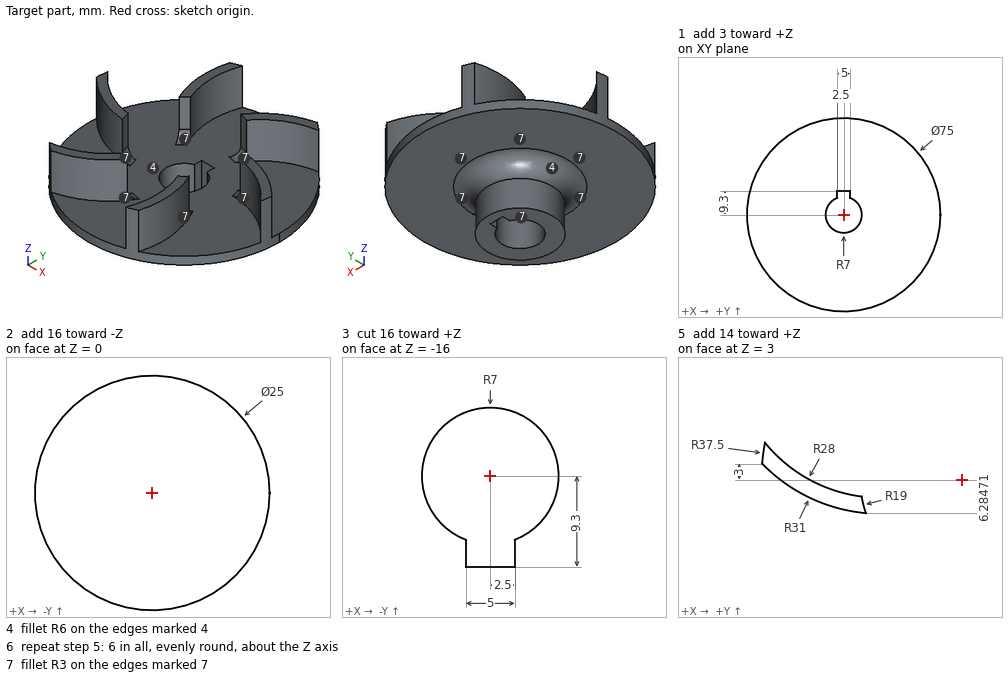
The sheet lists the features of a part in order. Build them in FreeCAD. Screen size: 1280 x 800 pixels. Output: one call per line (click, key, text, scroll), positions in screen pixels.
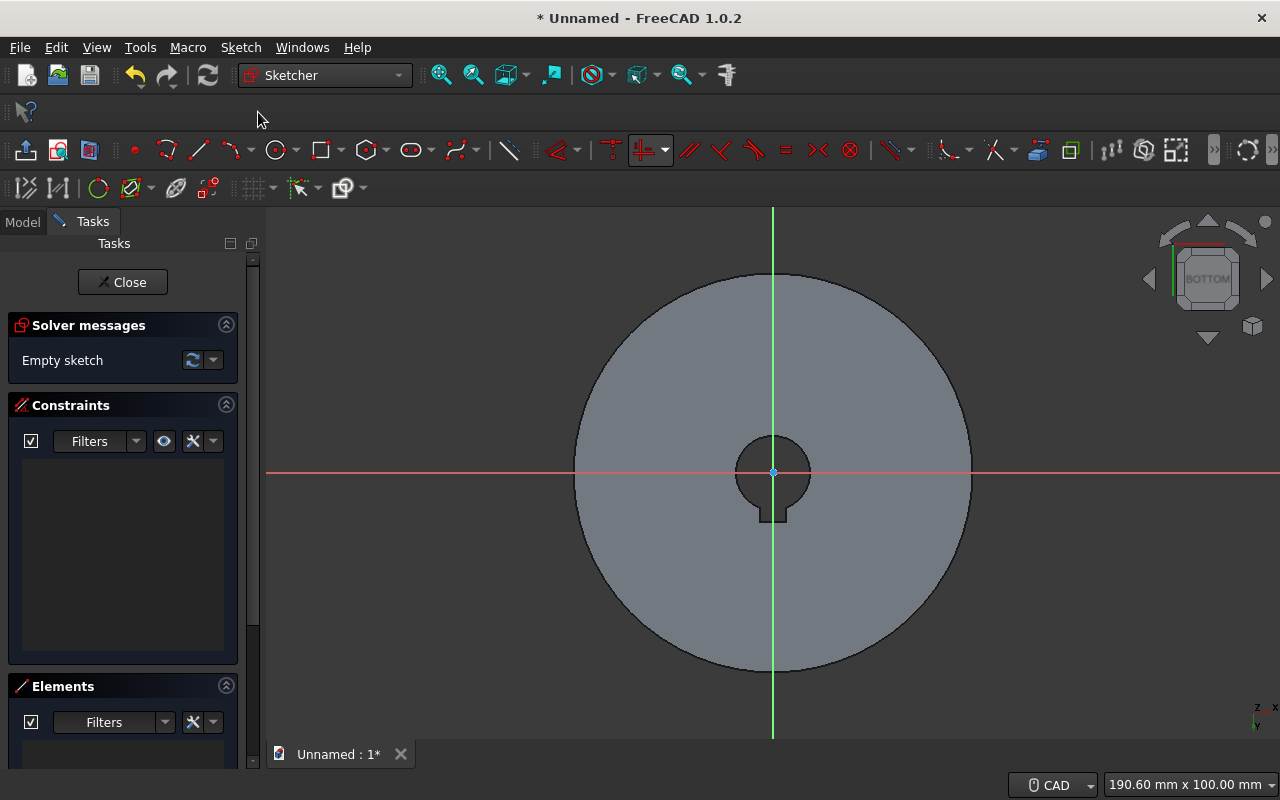
scroll(813, 473, up, 5)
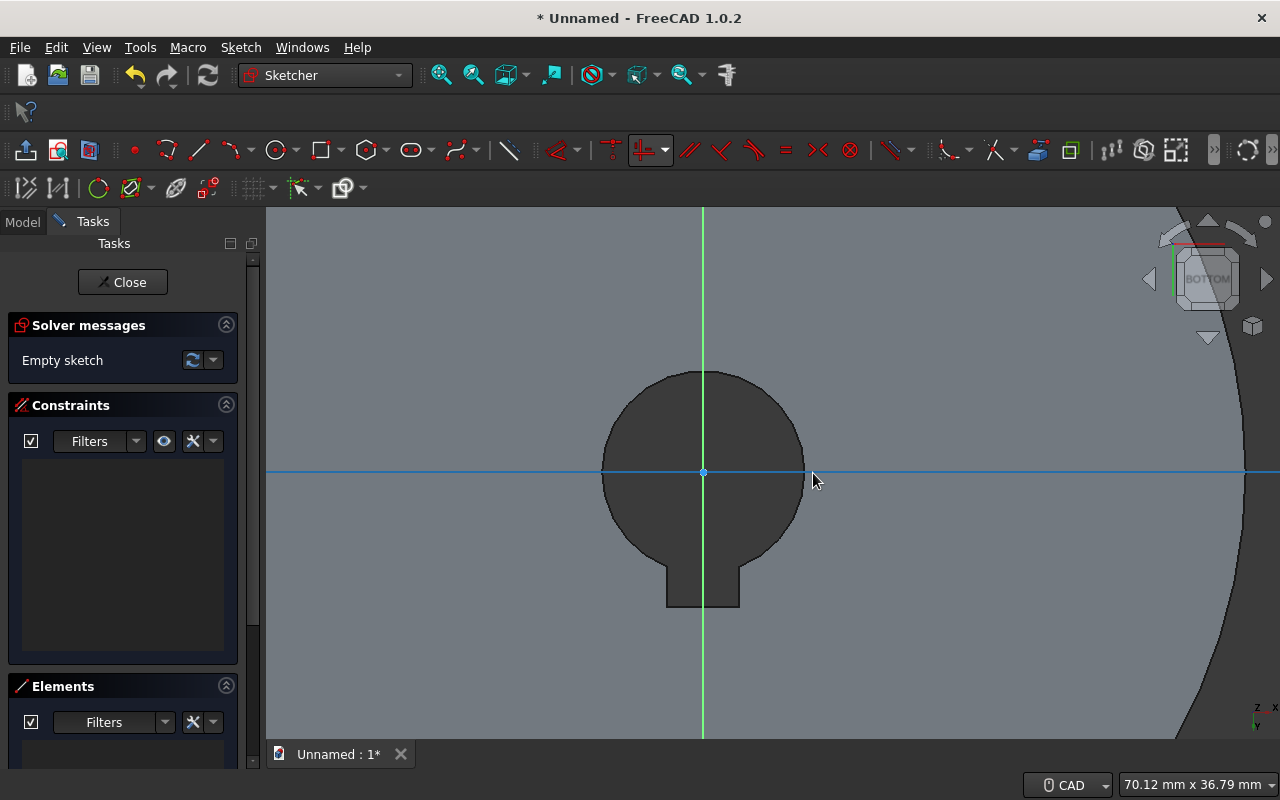
click(276, 150)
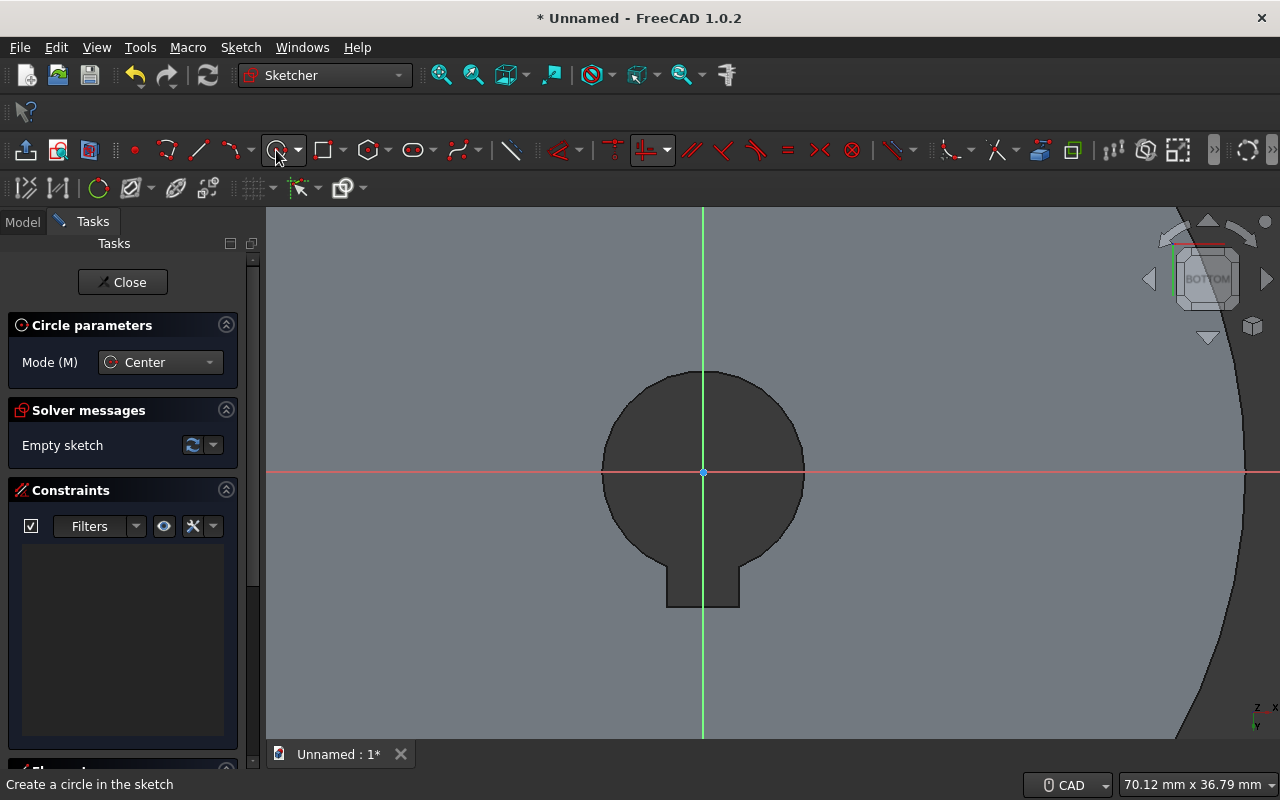
click(703, 472)
click(831, 344)
key(Escape)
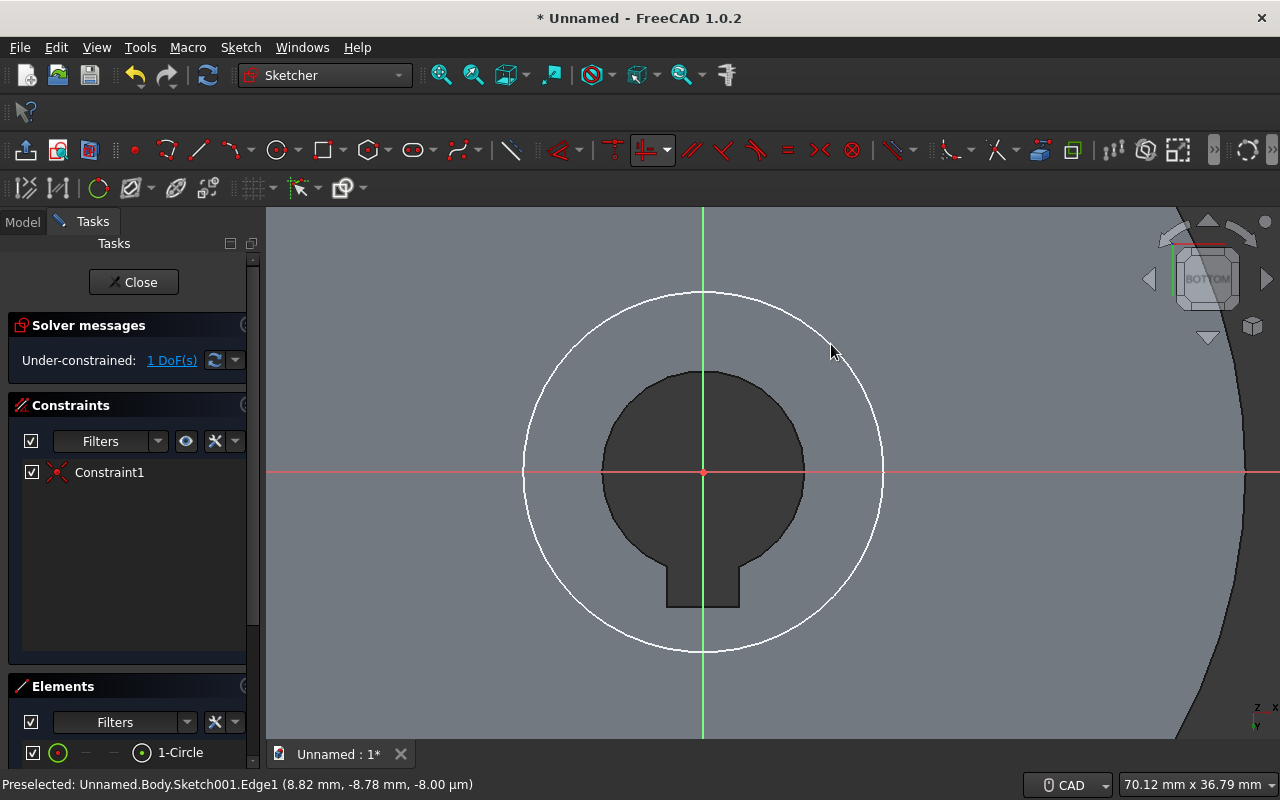
click(830, 344)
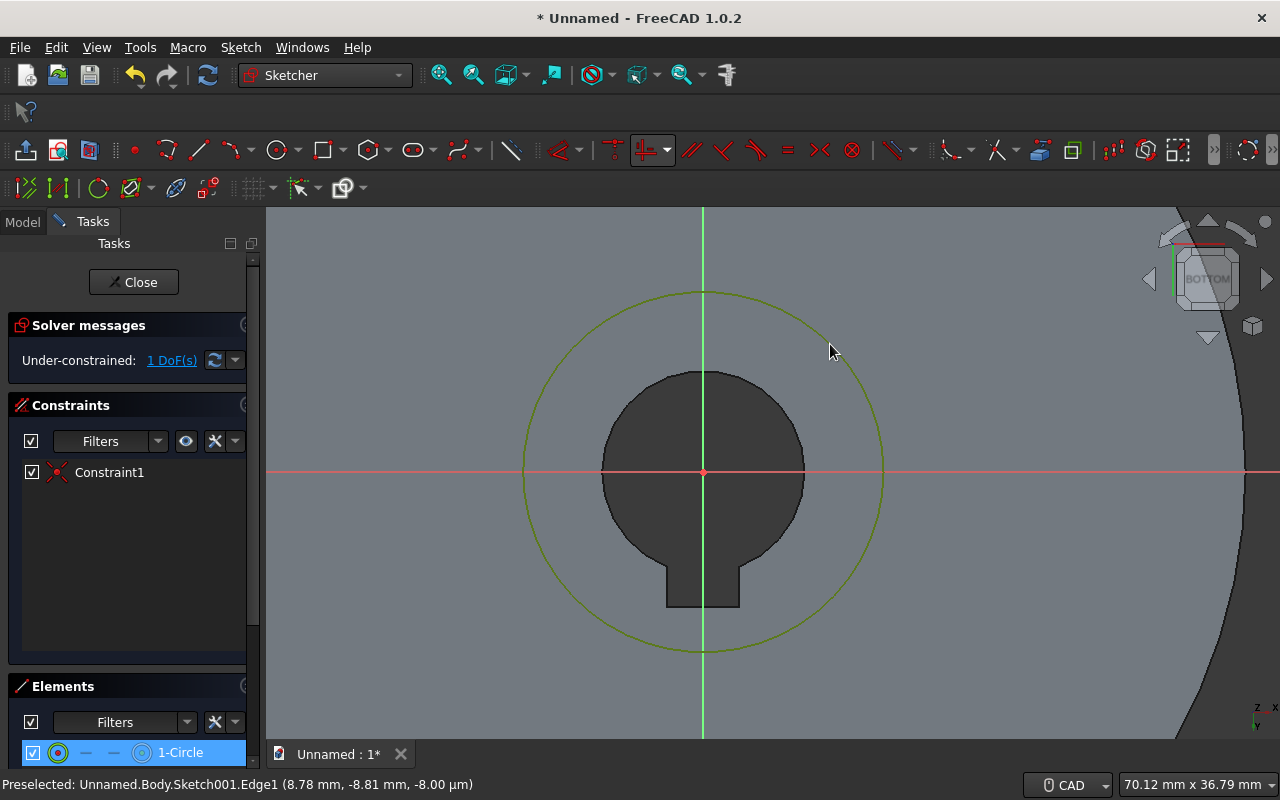
key(k)
key(o)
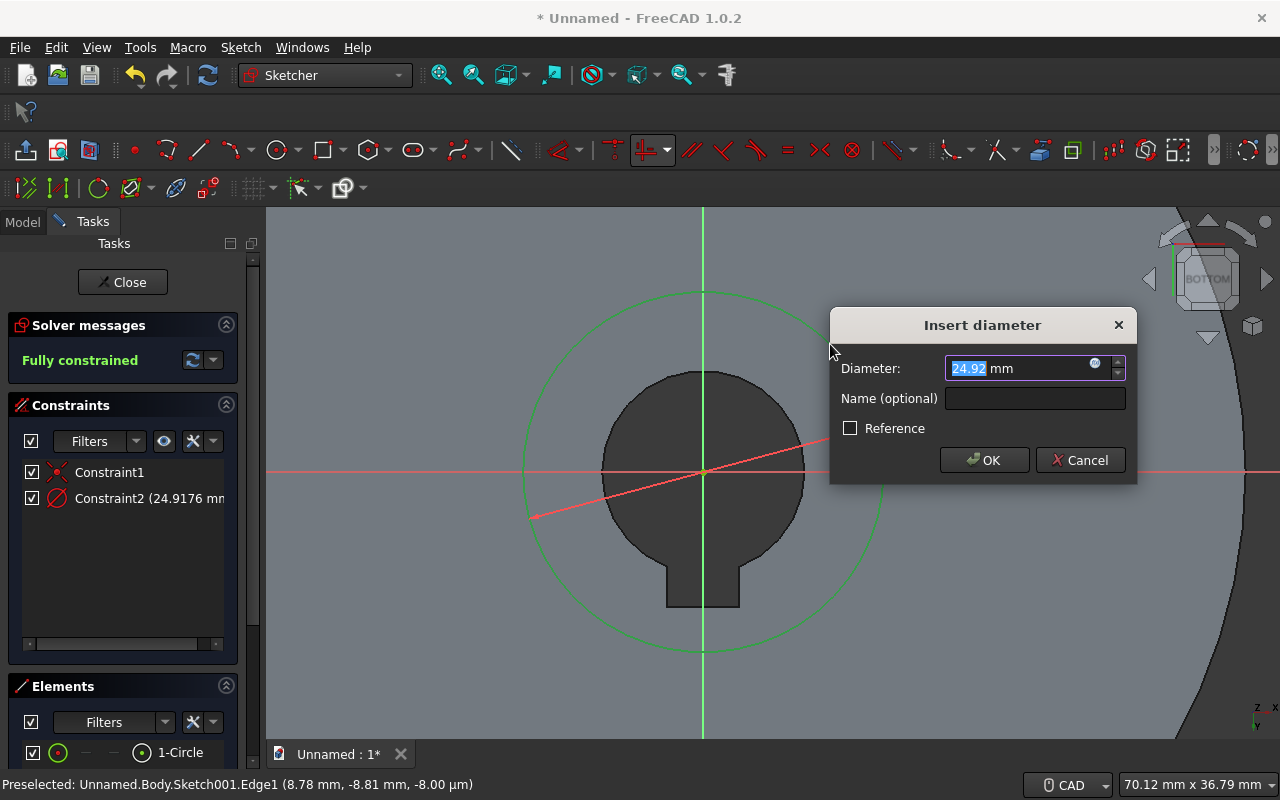
text(25)
key(Return)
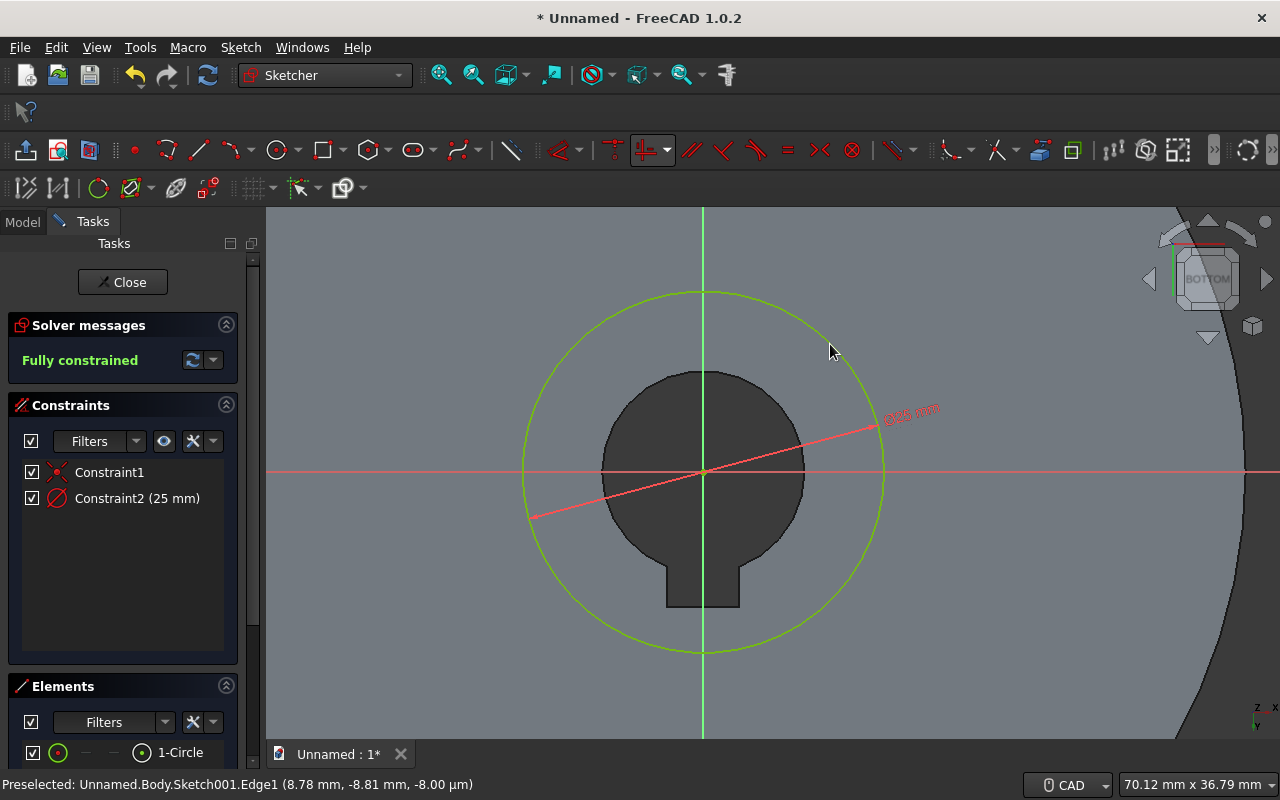
click(123, 282)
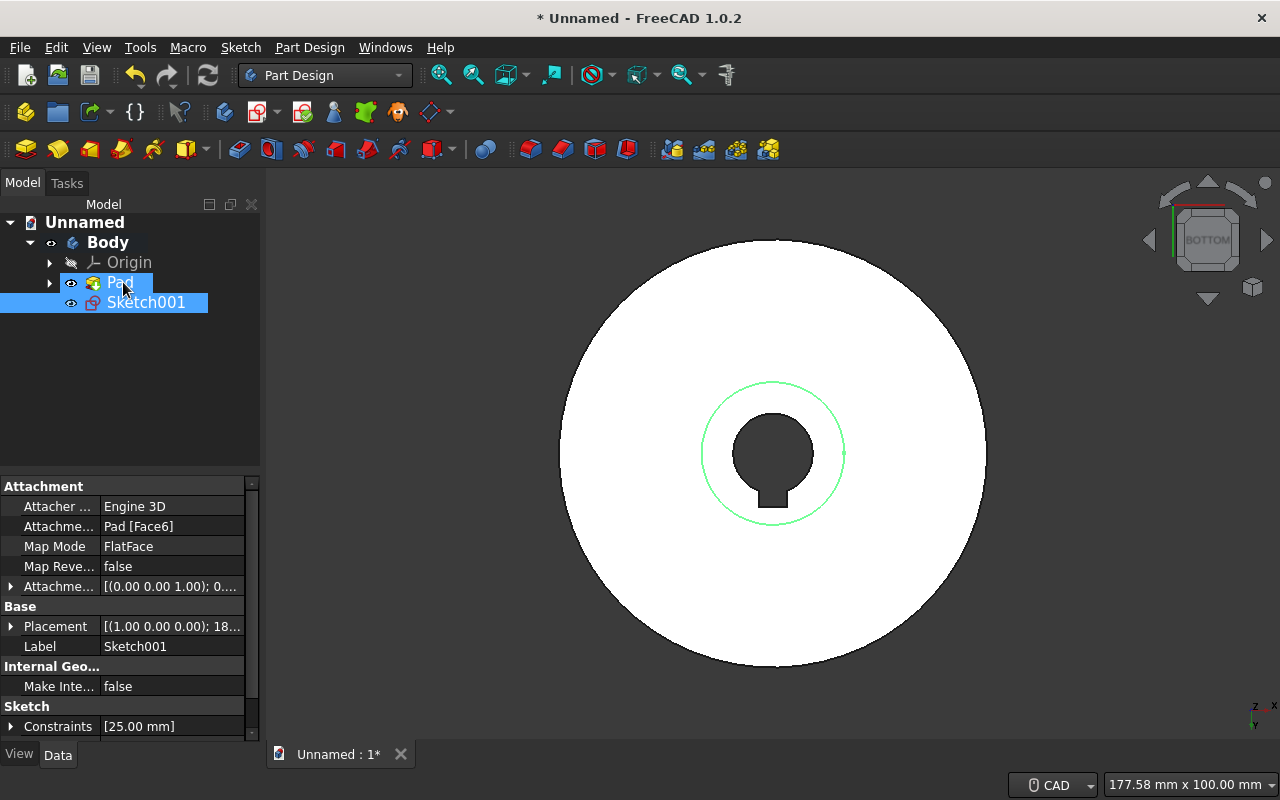
click(26, 150)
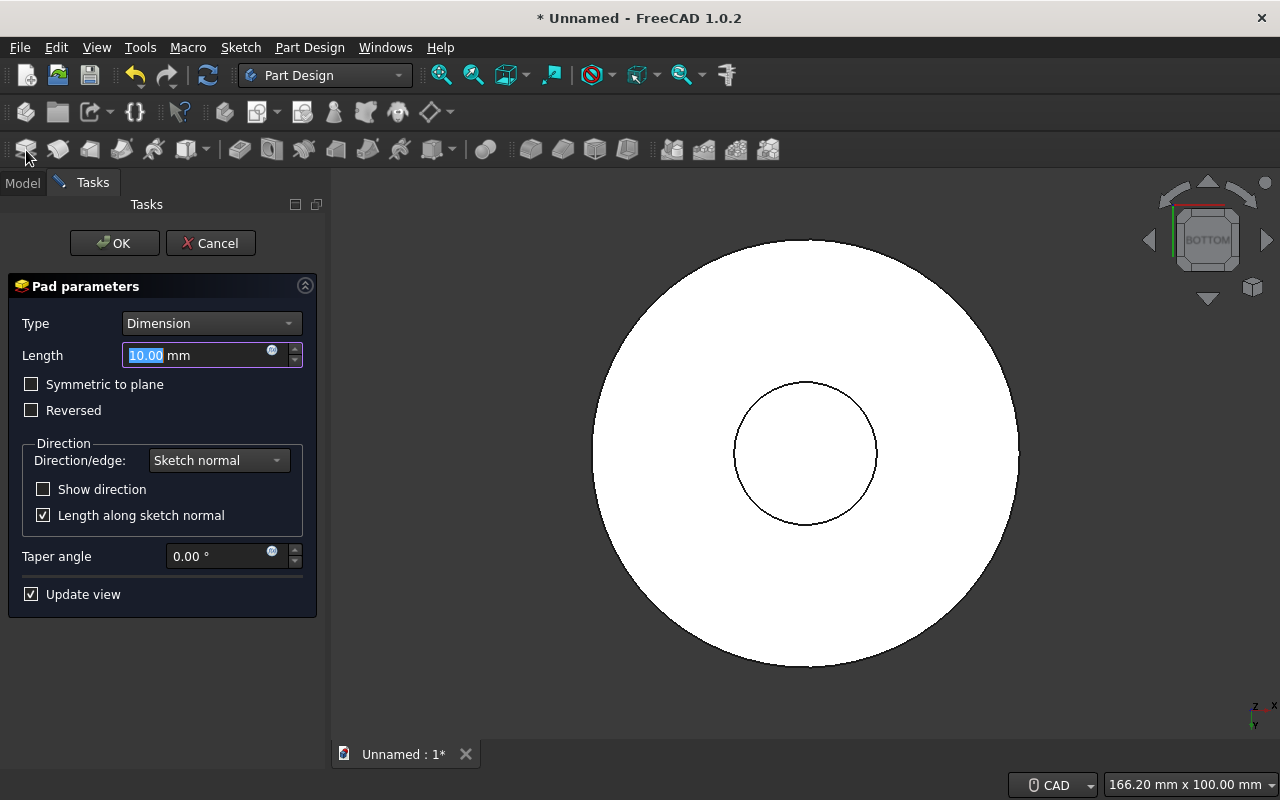
text(16)
key(Tab)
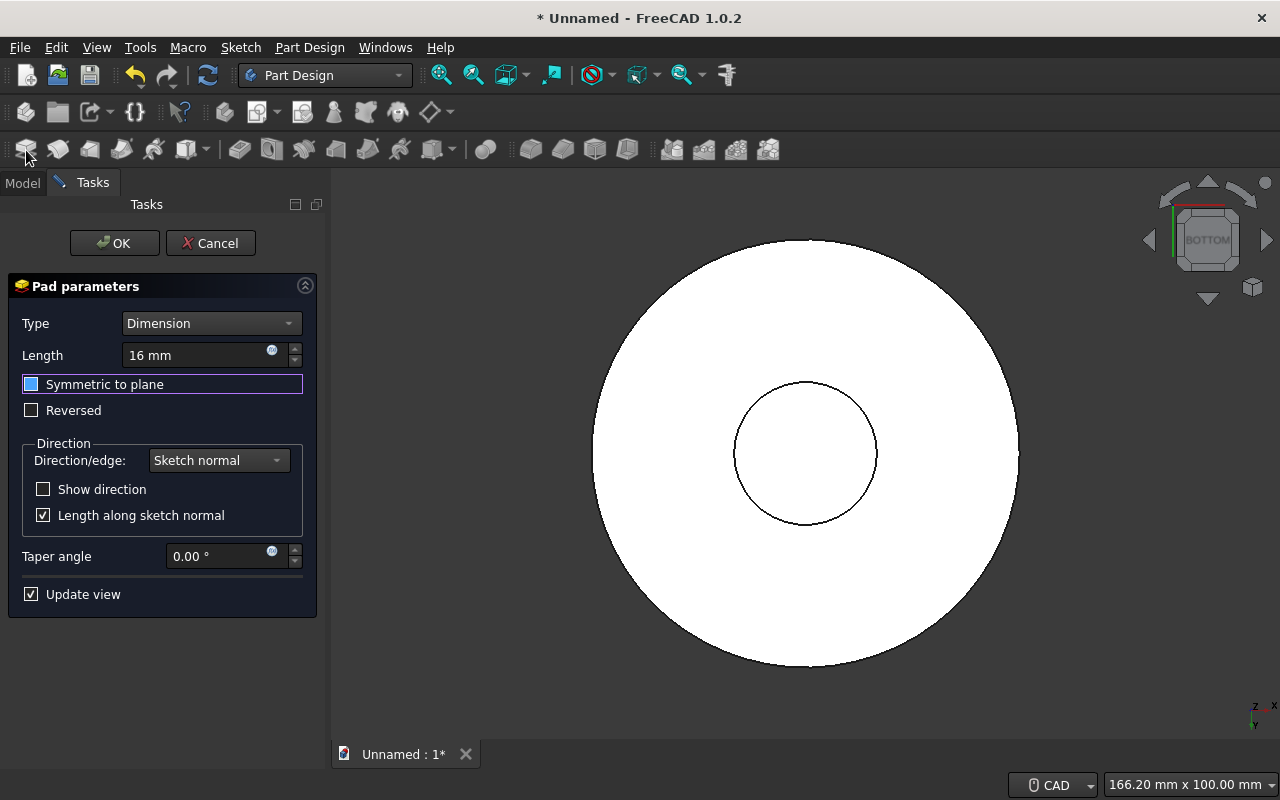
click(115, 243)